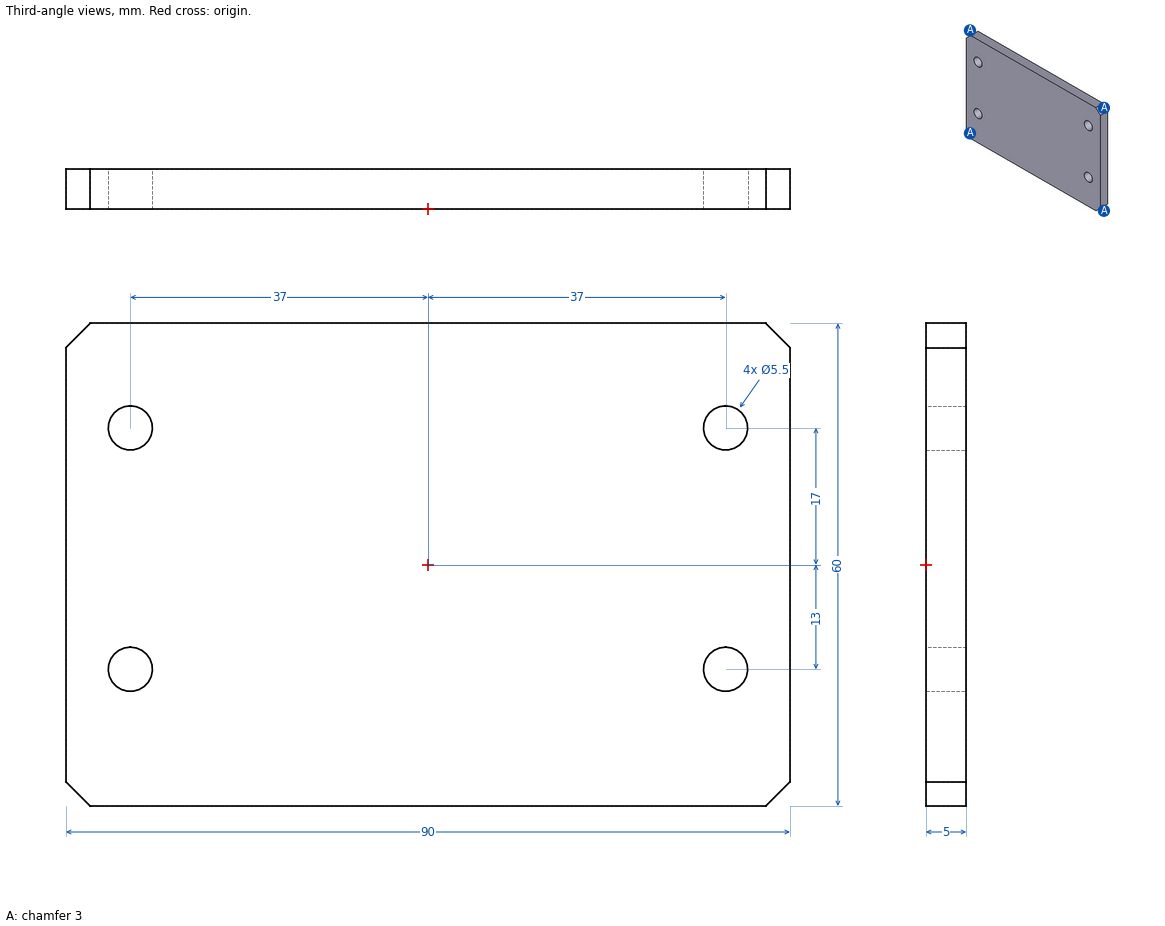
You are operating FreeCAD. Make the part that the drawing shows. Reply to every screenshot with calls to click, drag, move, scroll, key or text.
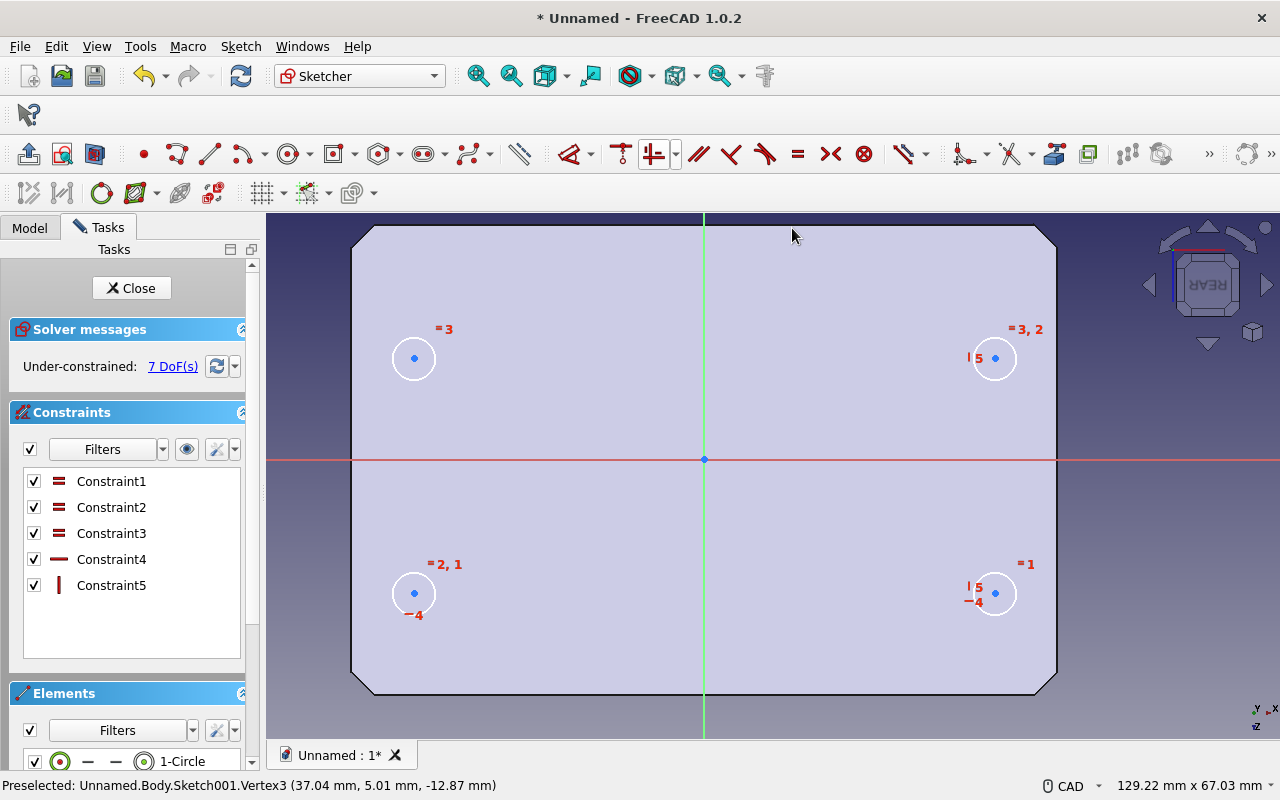
click(414, 594)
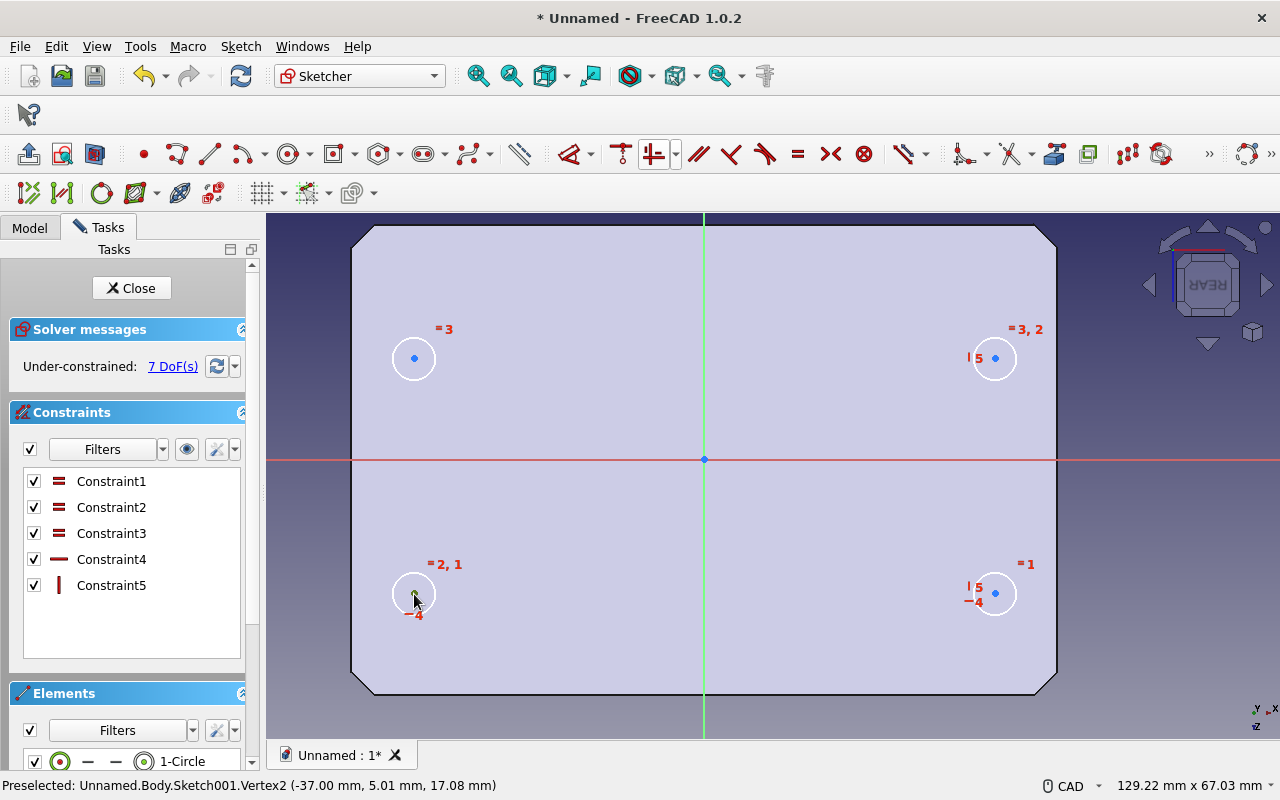
click(414, 359)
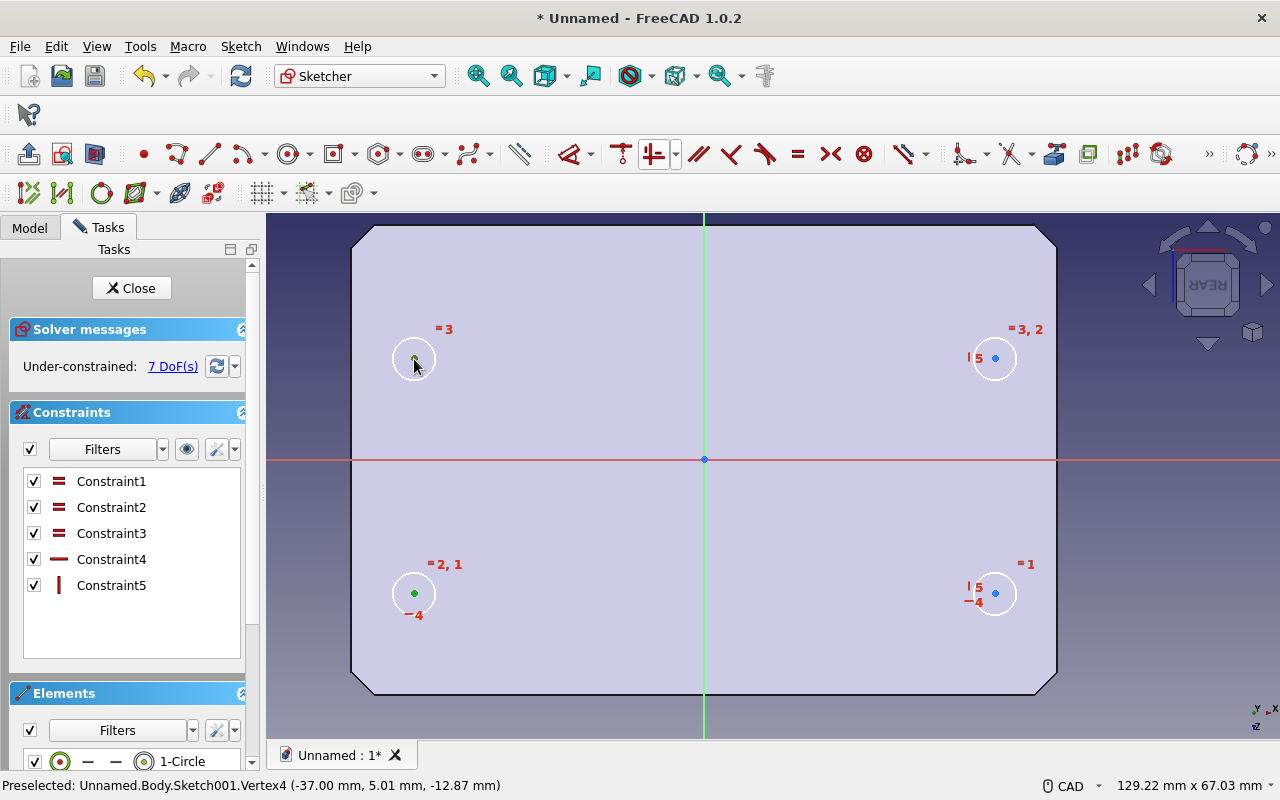
key(v)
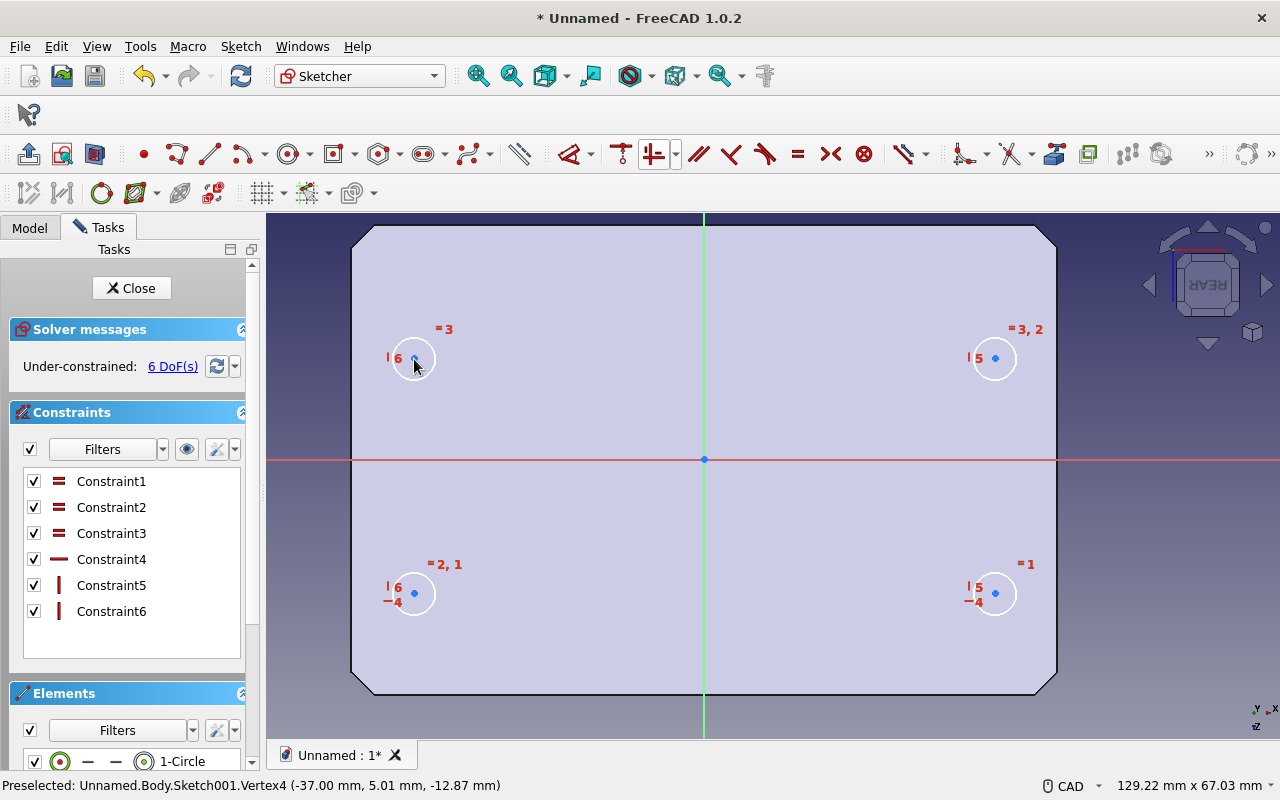
click(995, 359)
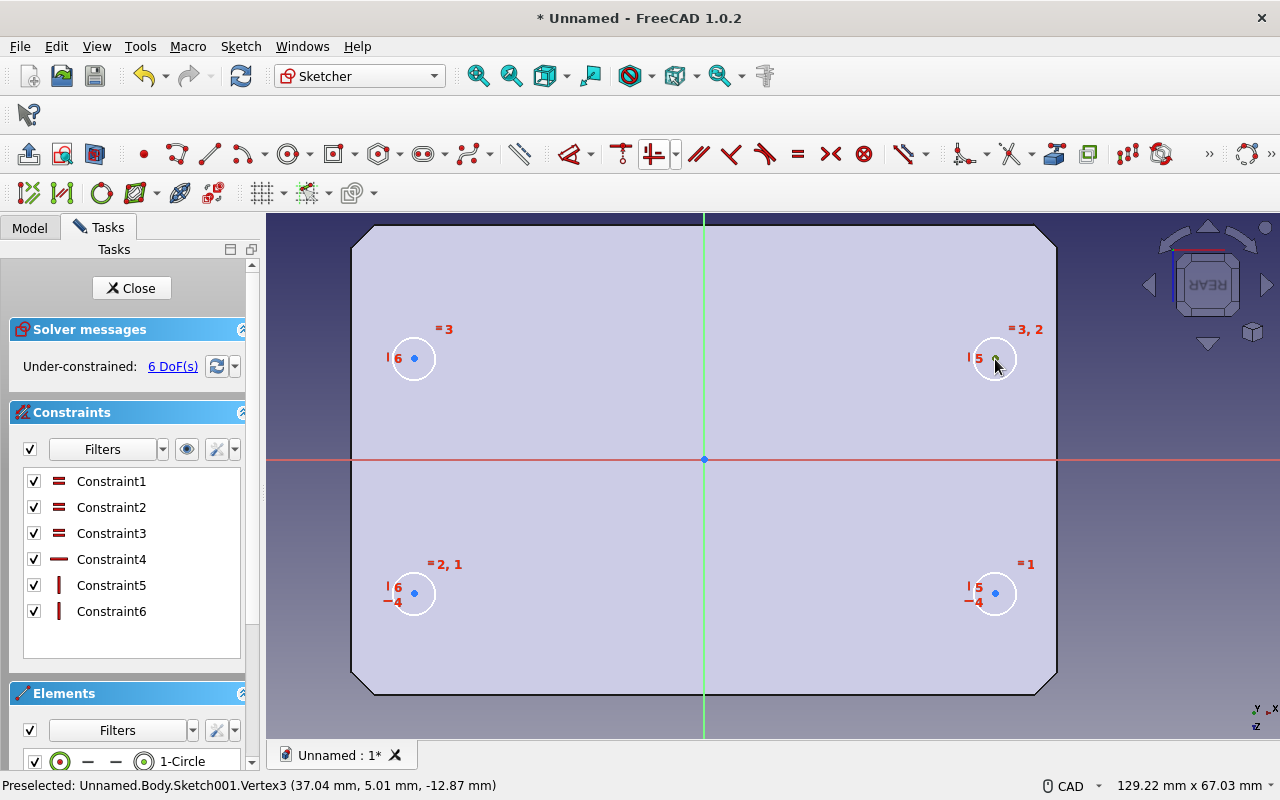
click(414, 359)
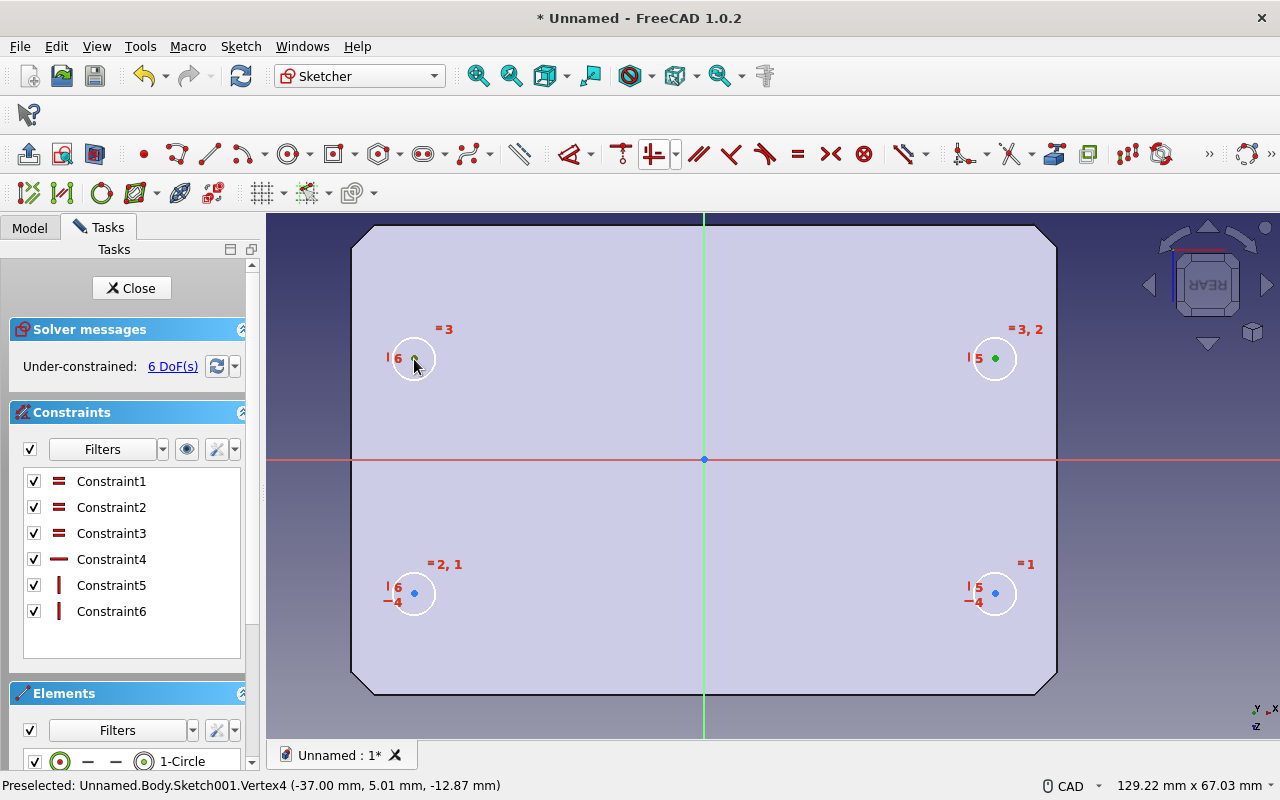
click(676, 154)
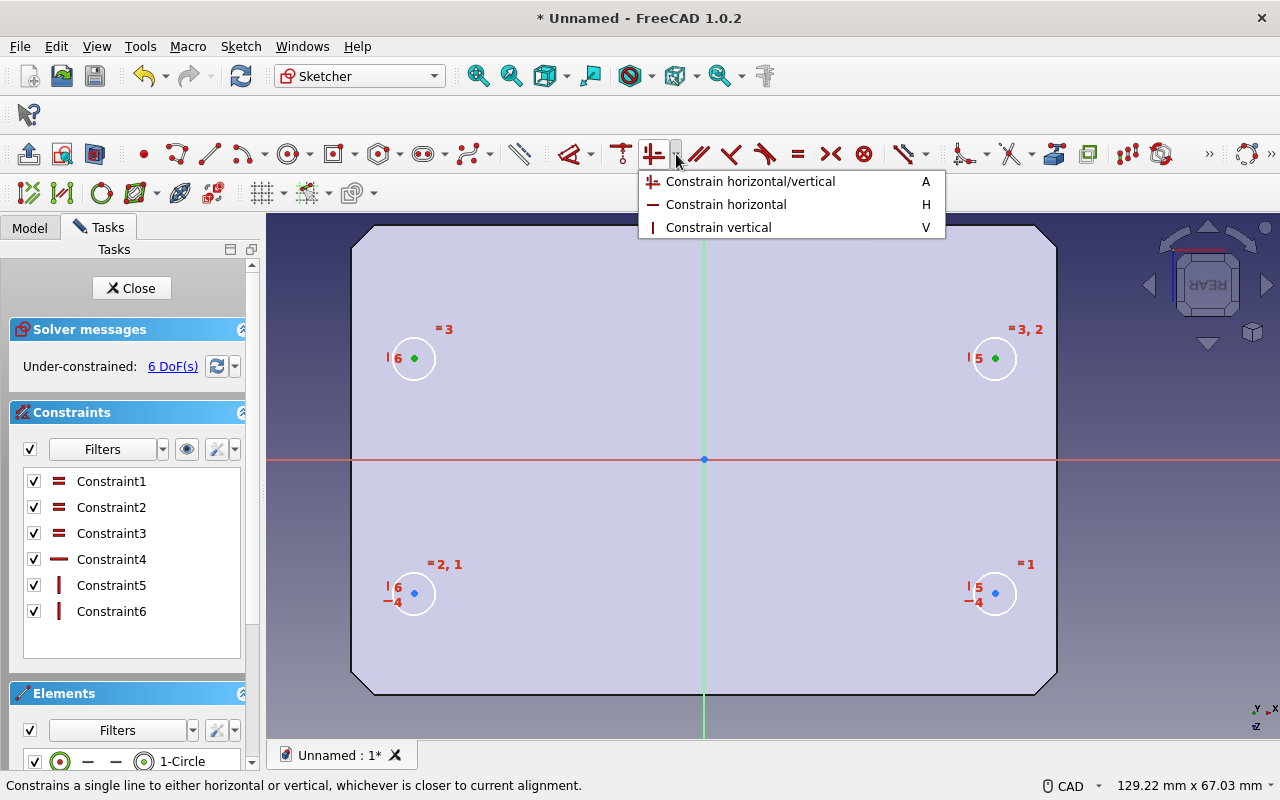
click(792, 204)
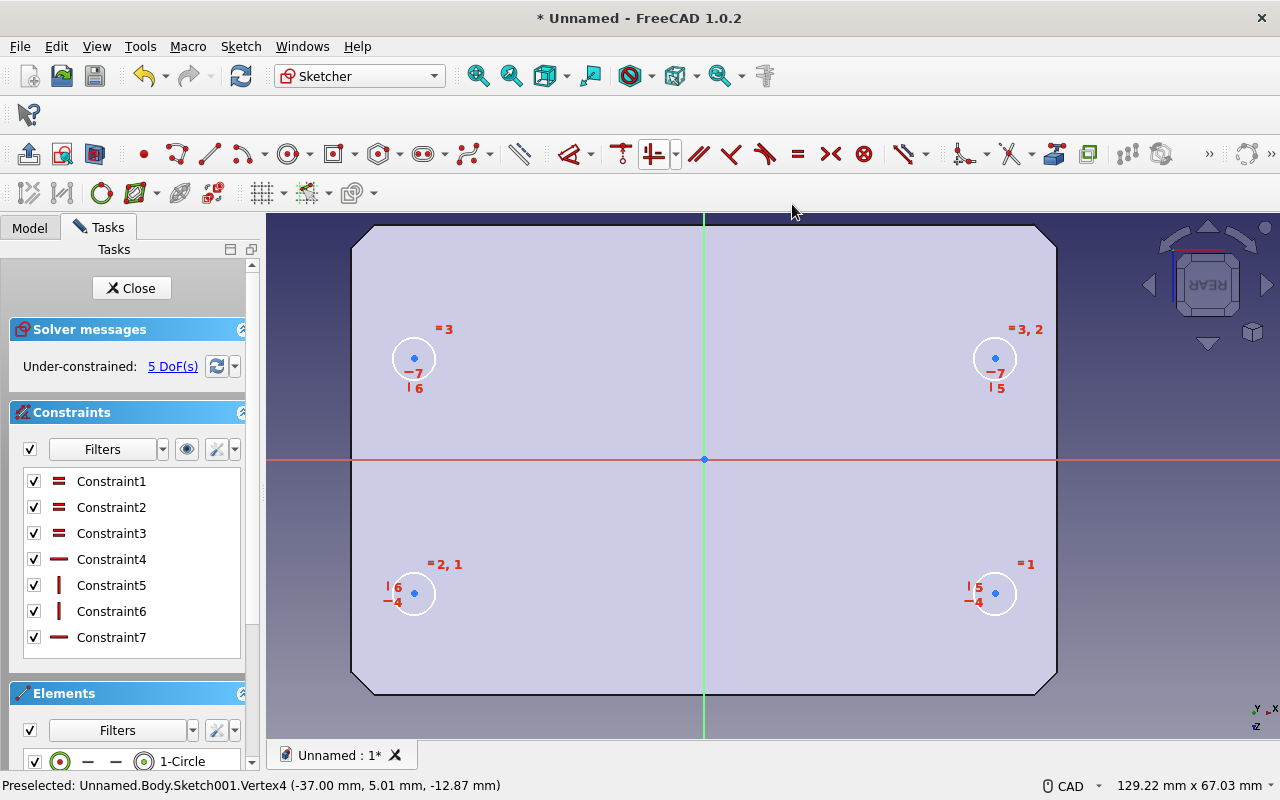
click(568, 154)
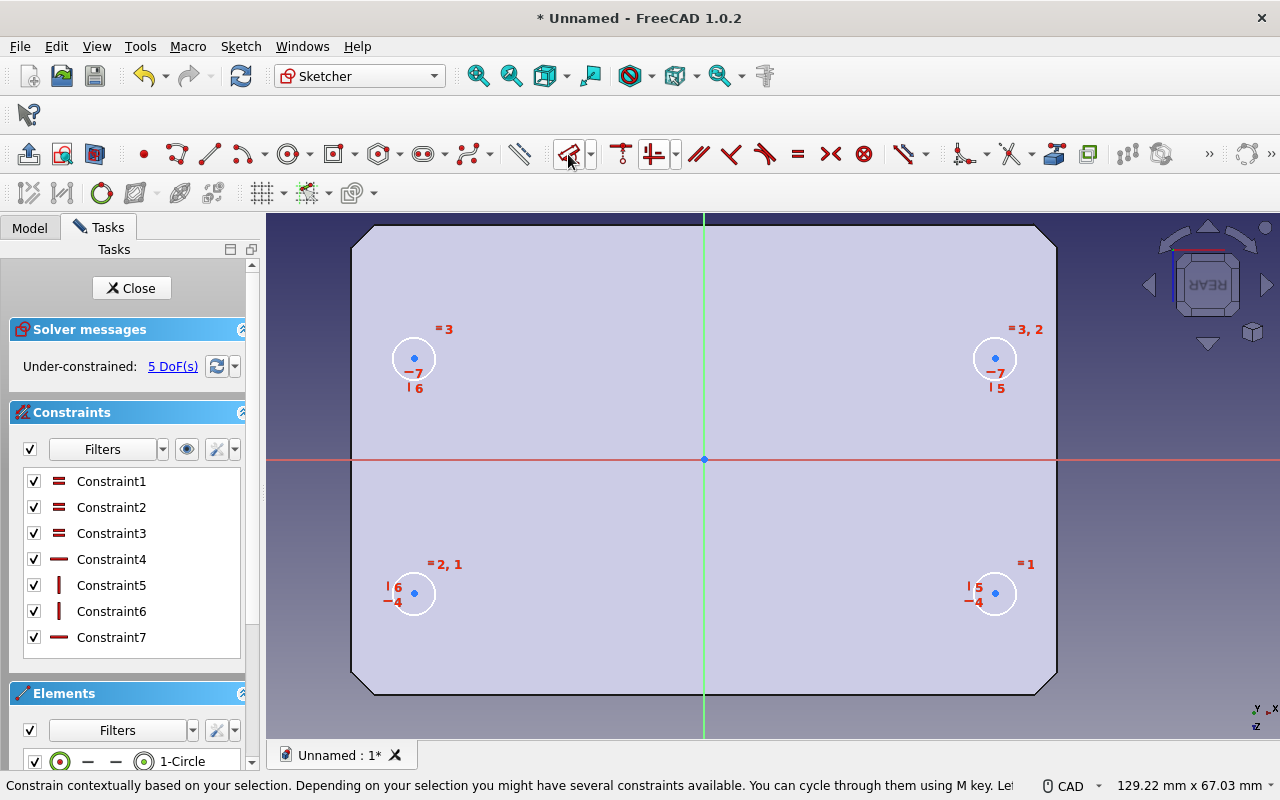
click(1010, 579)
click(1033, 556)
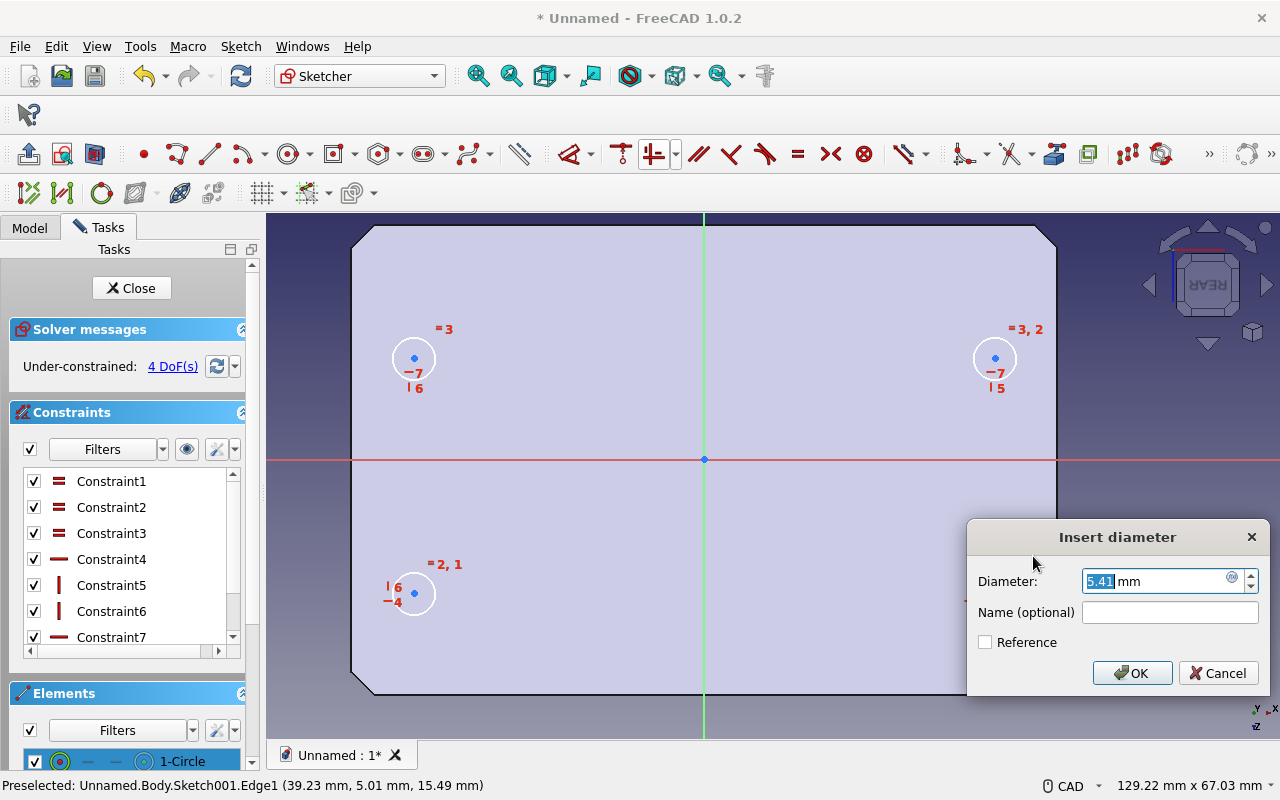
text(5.5)
key(Return)